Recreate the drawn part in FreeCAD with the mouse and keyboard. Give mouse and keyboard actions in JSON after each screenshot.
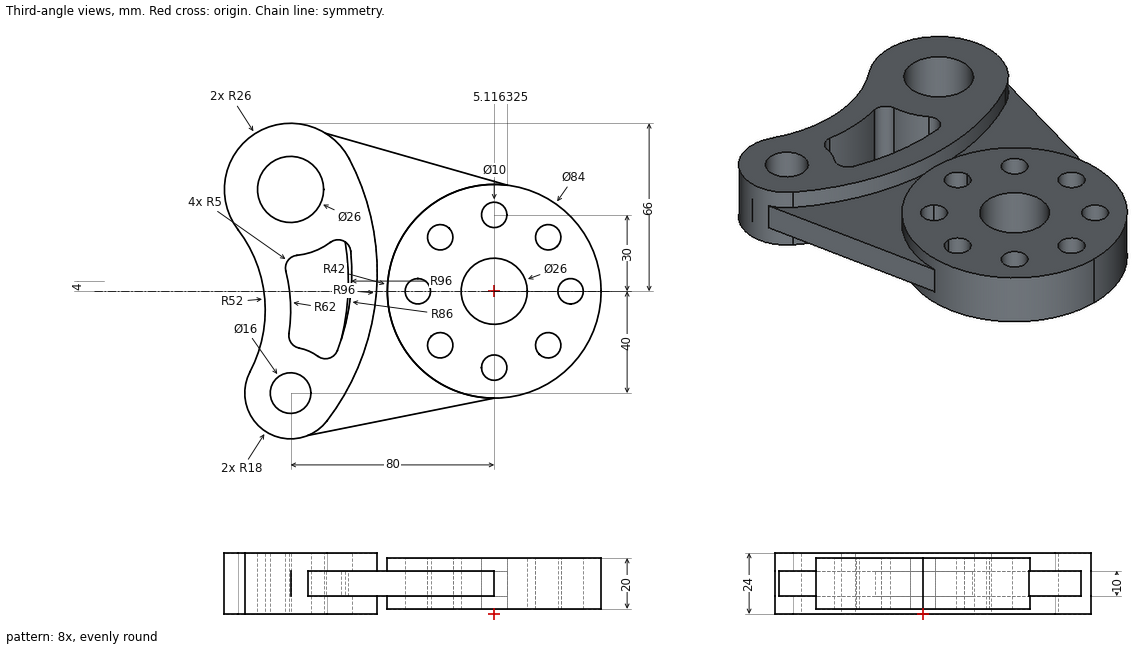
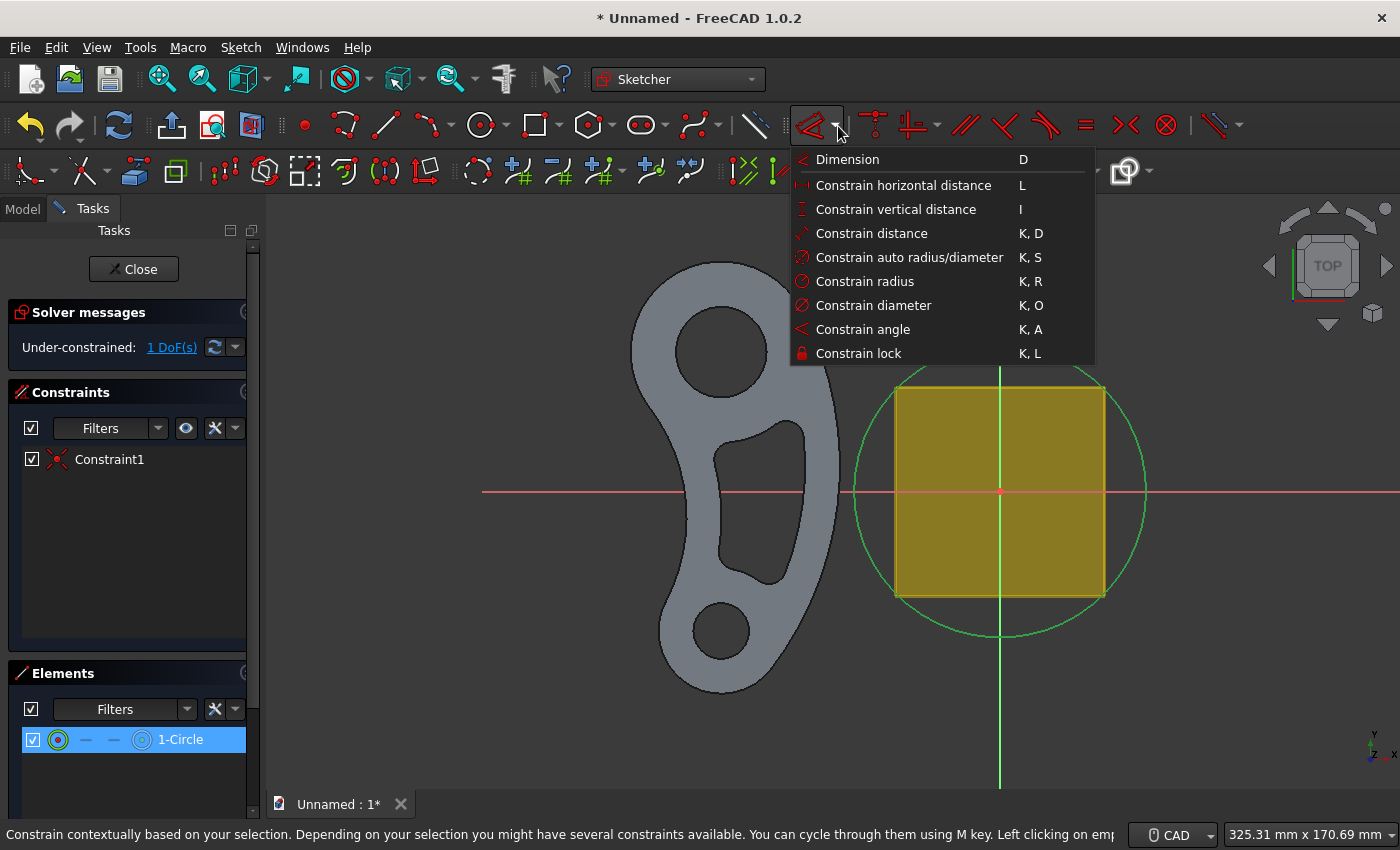
{"action": "left_click", "coordinate": [943, 305]}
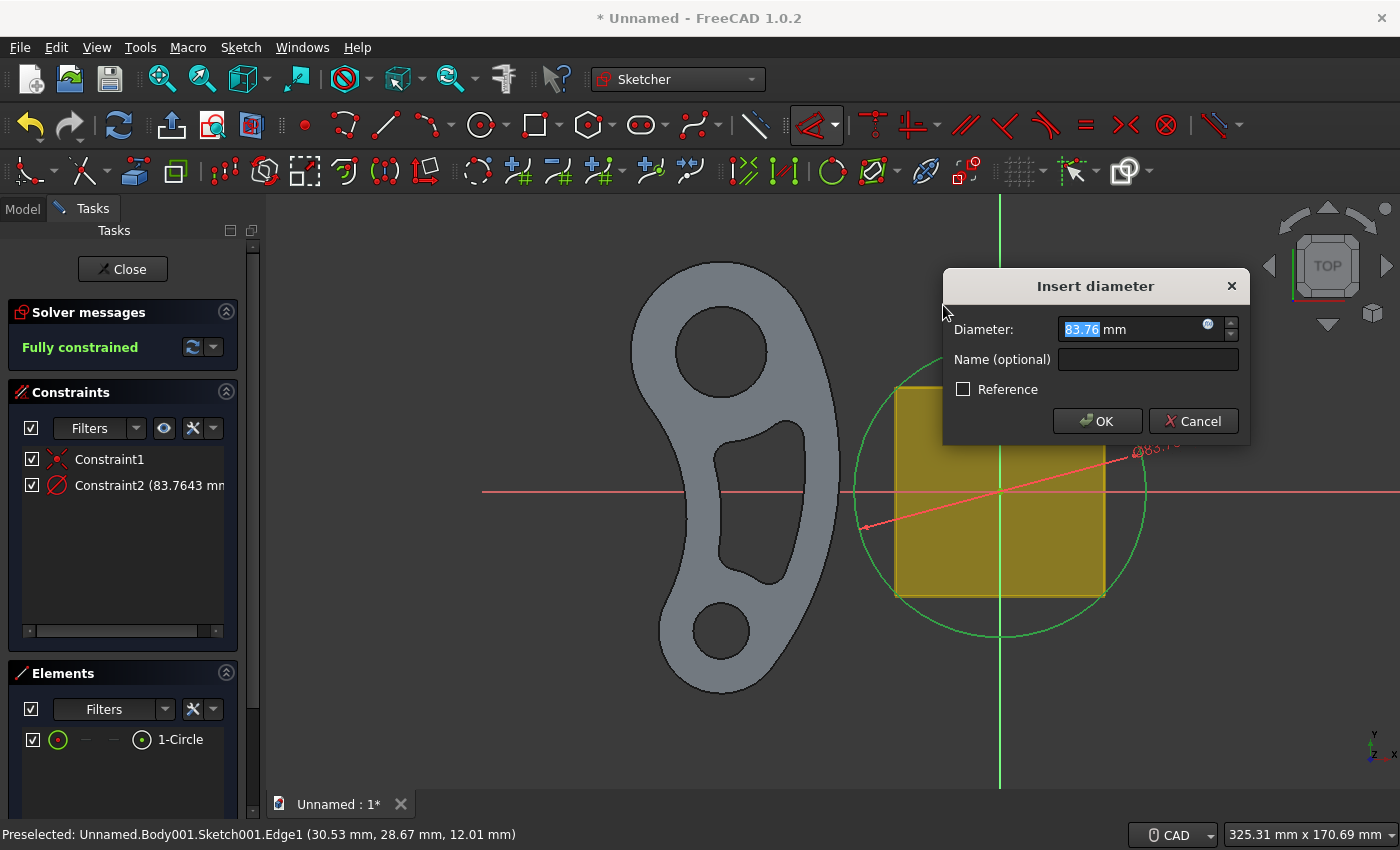
{"action": "type", "text": "84"}
{"action": "key", "text": "Return"}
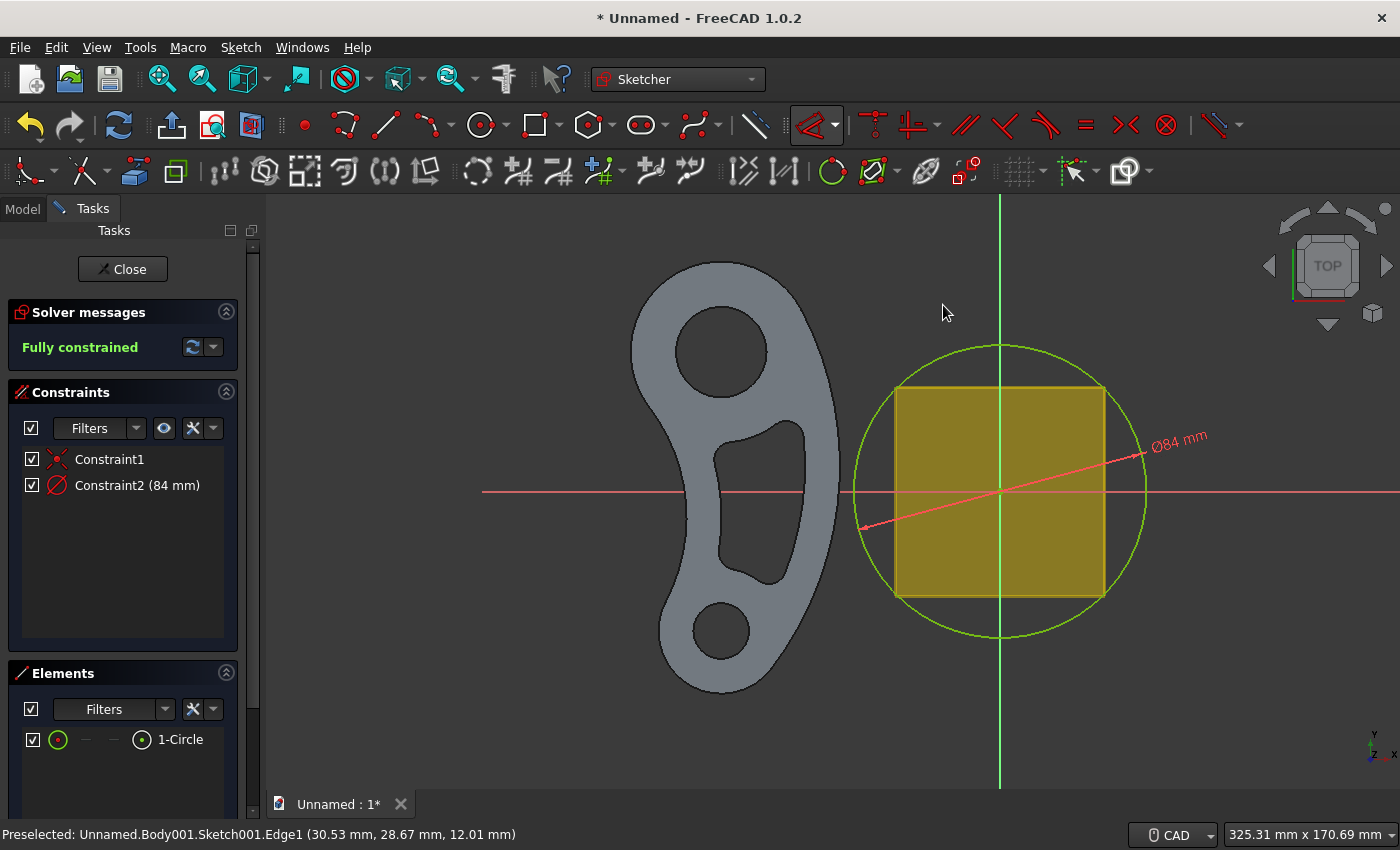
{"action": "left_click", "coordinate": [123, 269]}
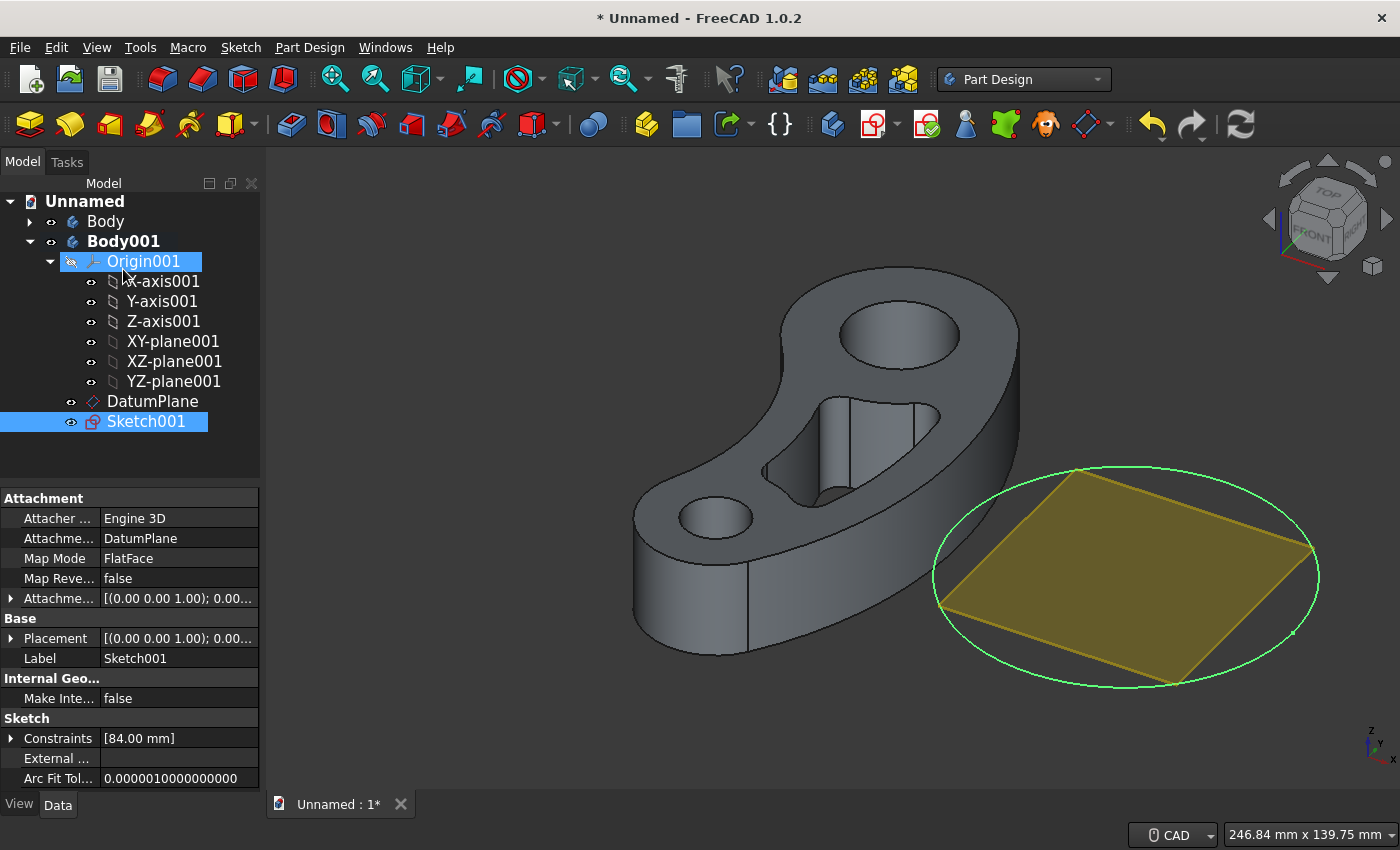
{"action": "left_click", "coordinate": [30, 124]}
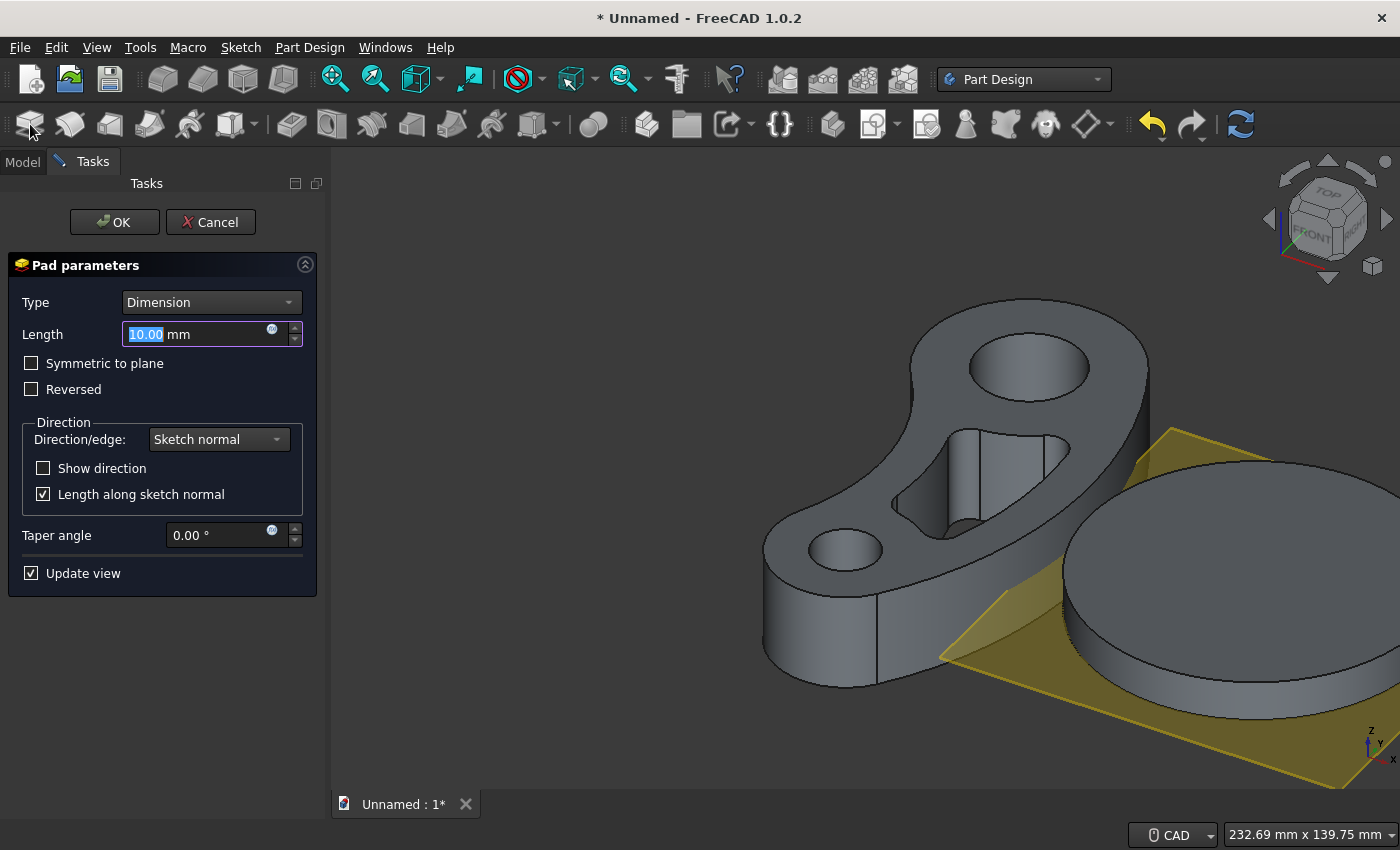
{"action": "type", "text": "20"}
{"action": "key", "text": "Tab"}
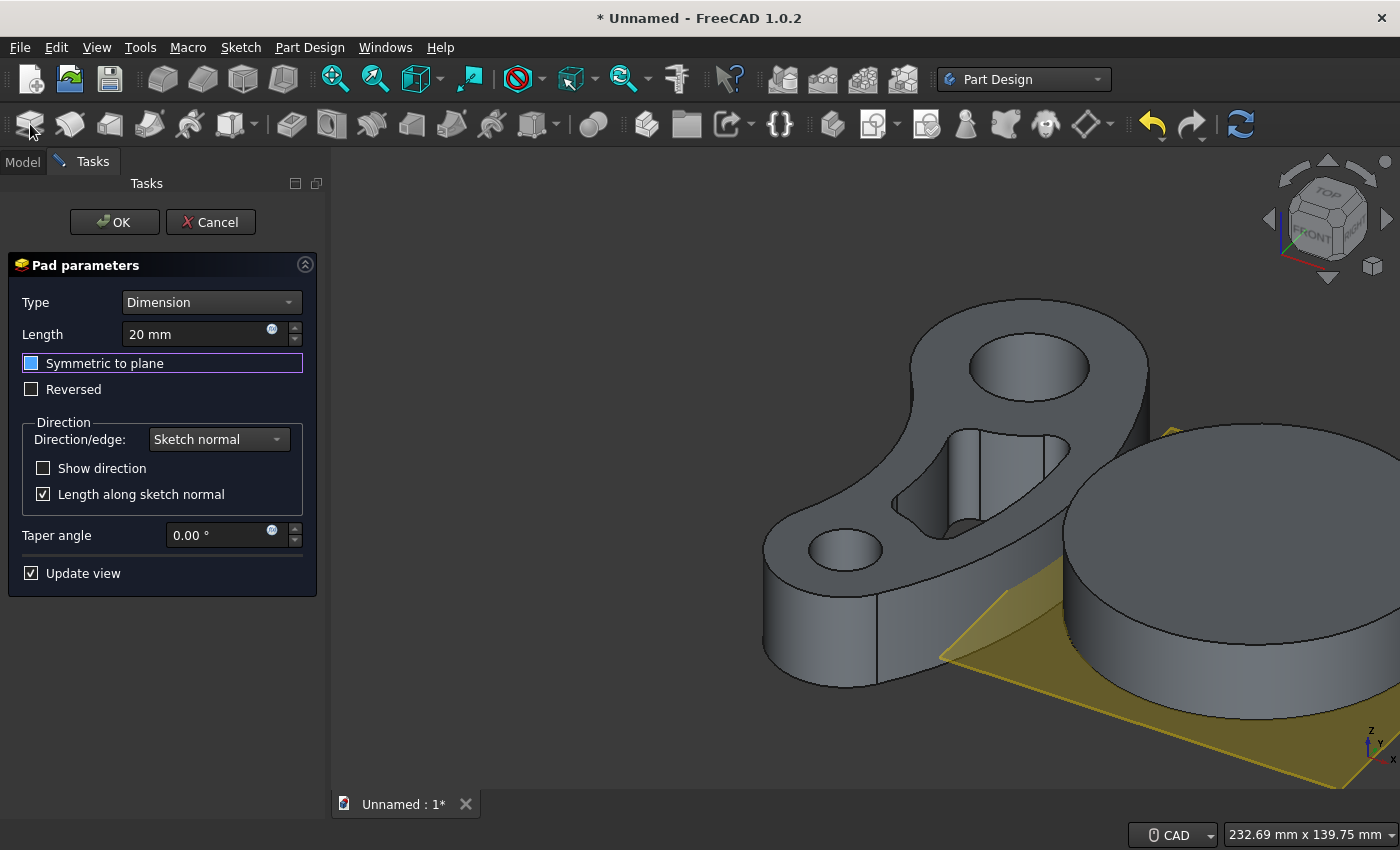
{"action": "left_click", "coordinate": [30, 363]}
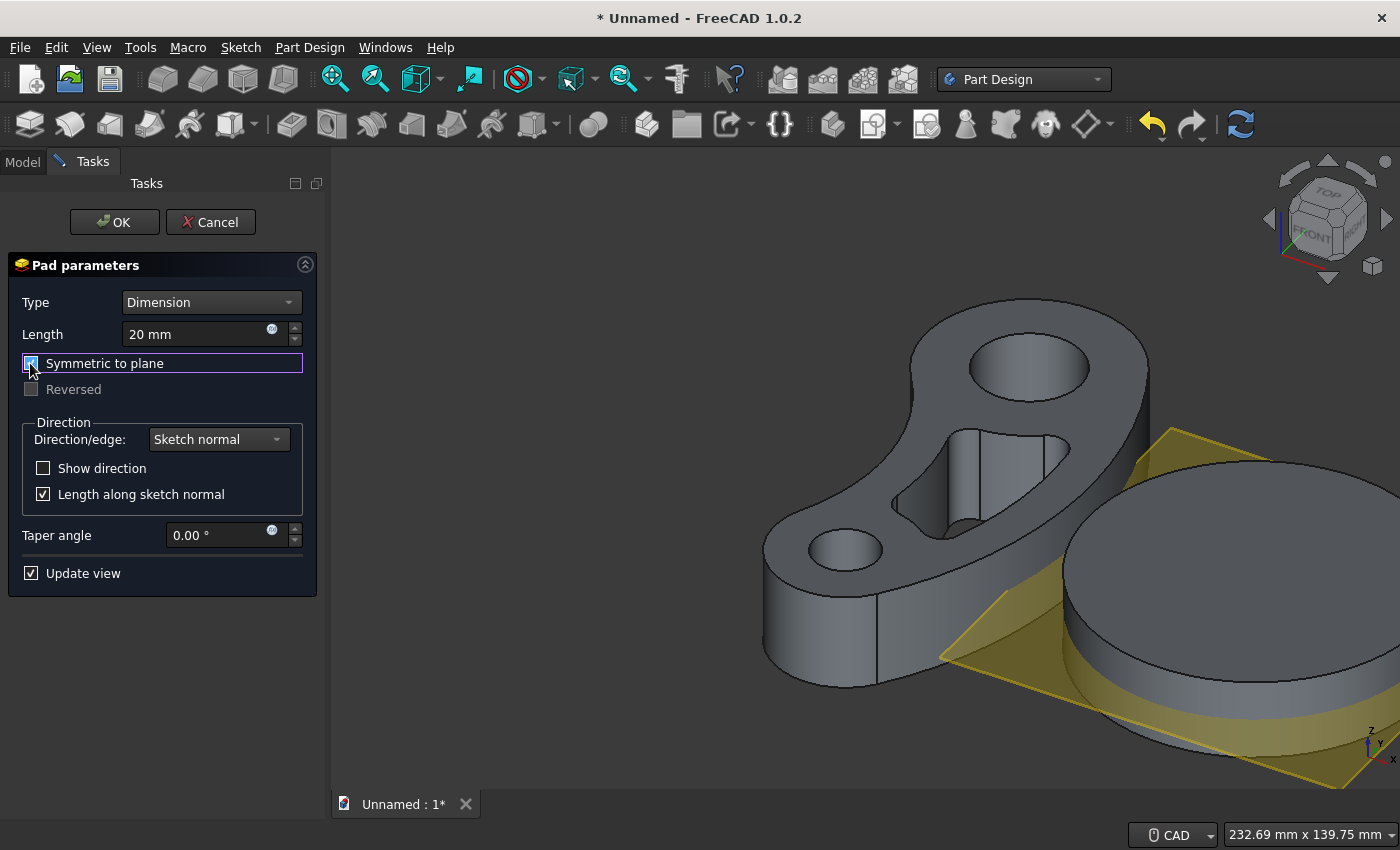
{"action": "left_click", "coordinate": [115, 222]}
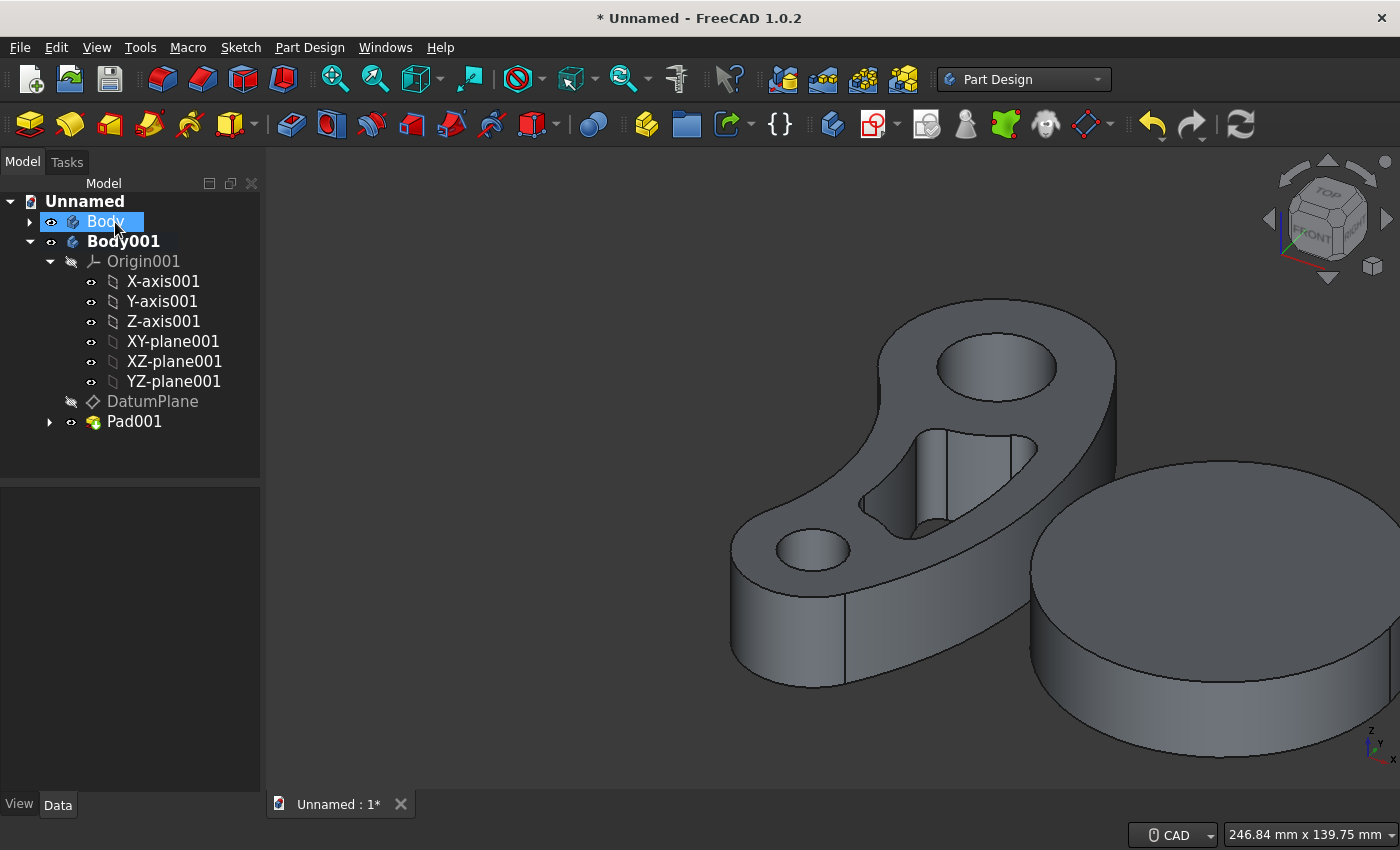
{"action": "left_click", "coordinate": [336, 80]}